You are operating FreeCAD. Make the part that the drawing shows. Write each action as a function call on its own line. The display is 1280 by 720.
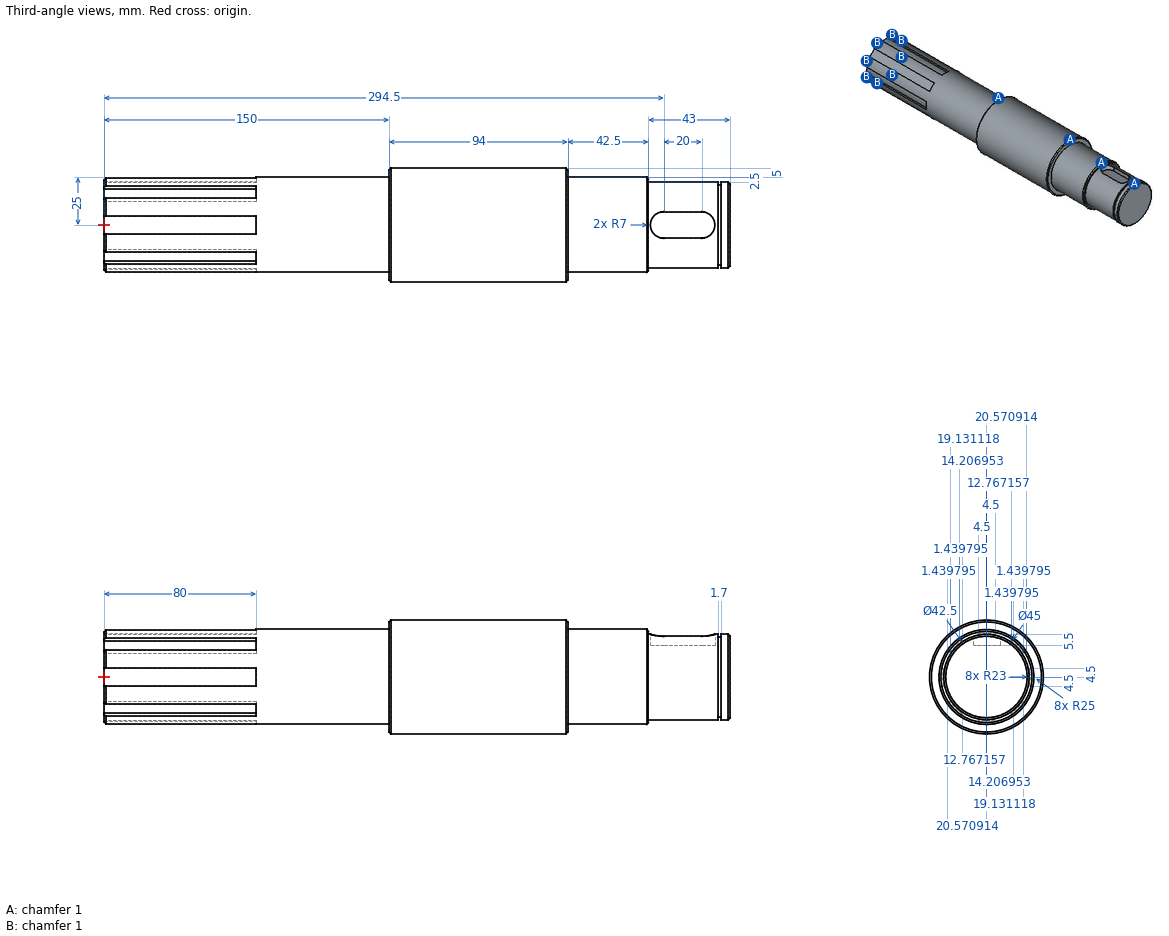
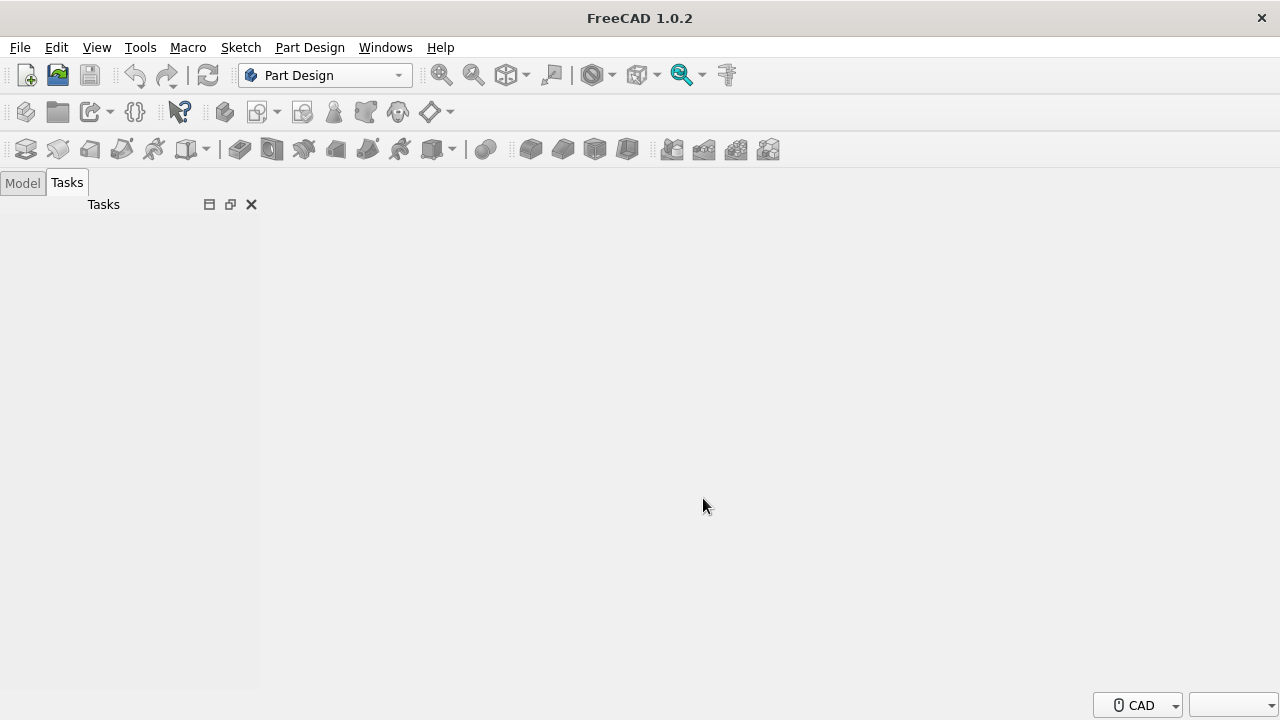
click(26, 76)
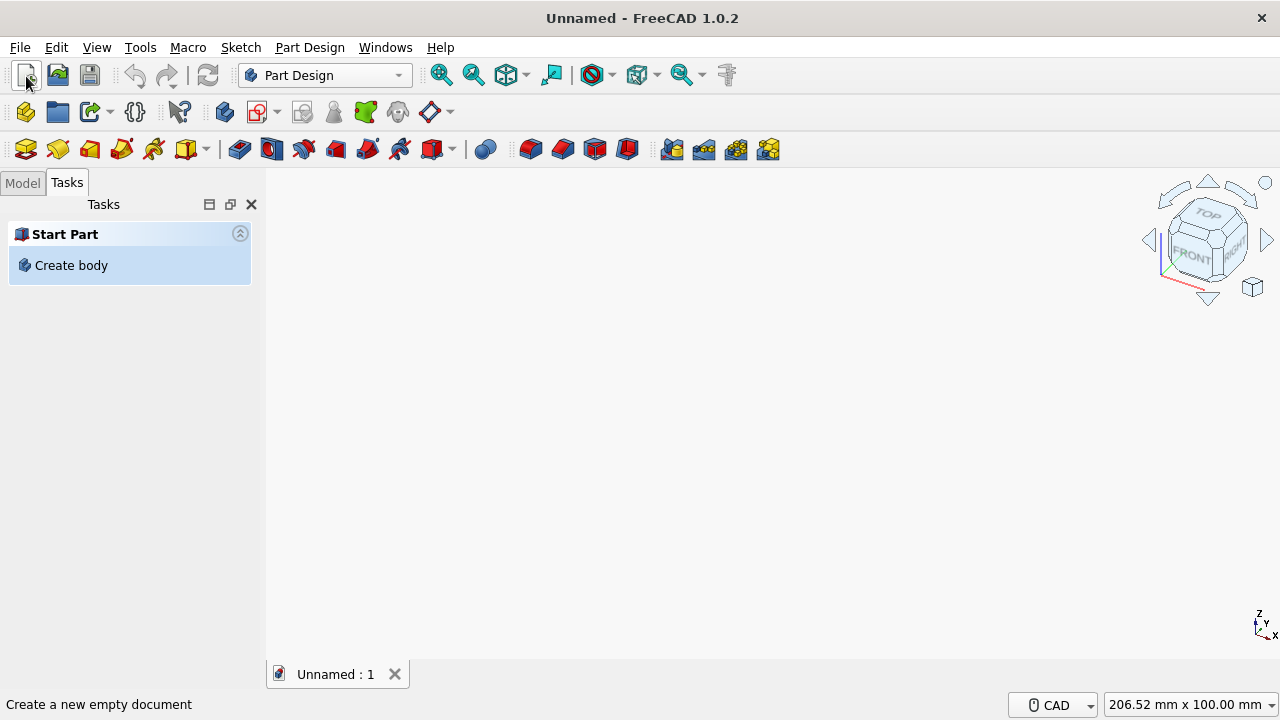
click(258, 112)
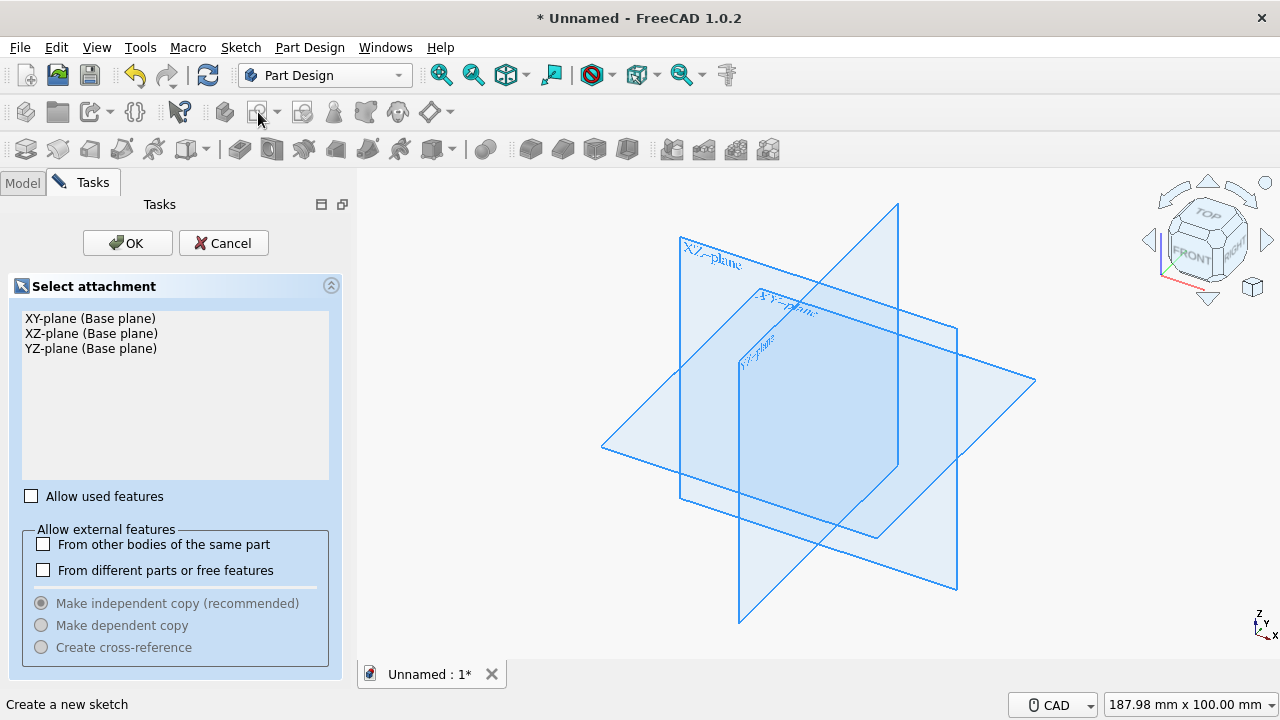
click(82, 318)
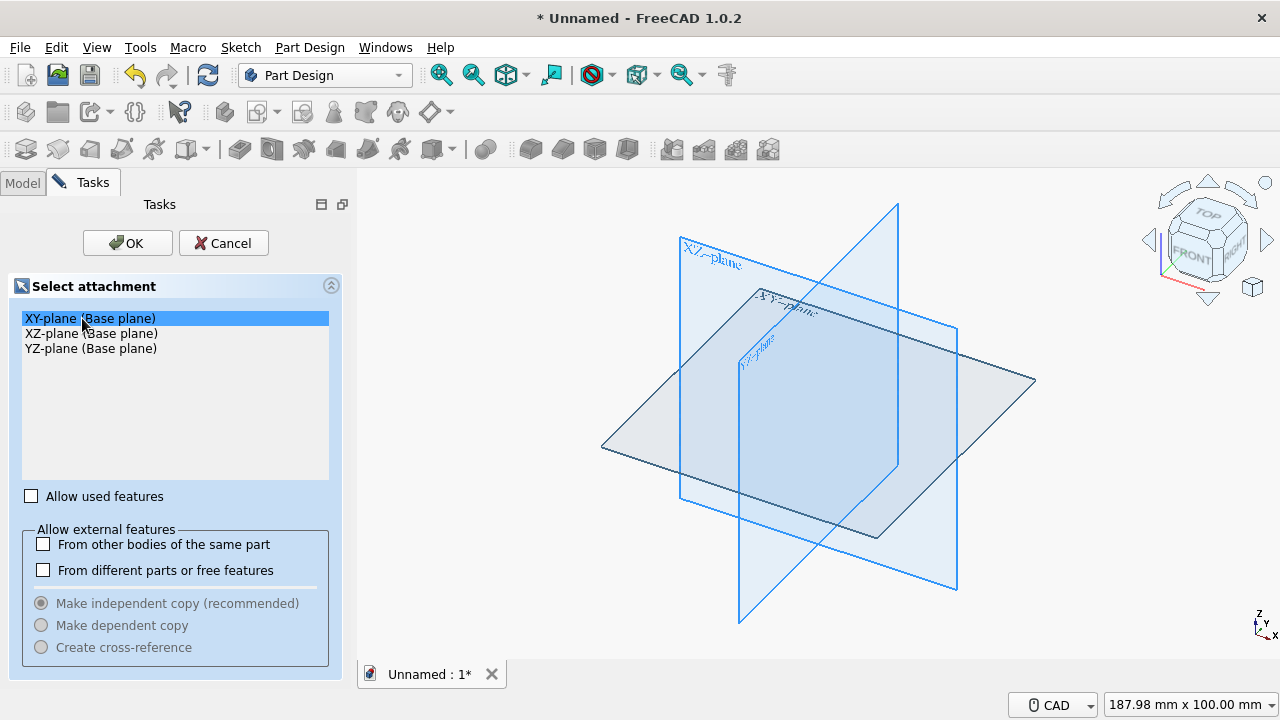
click(128, 243)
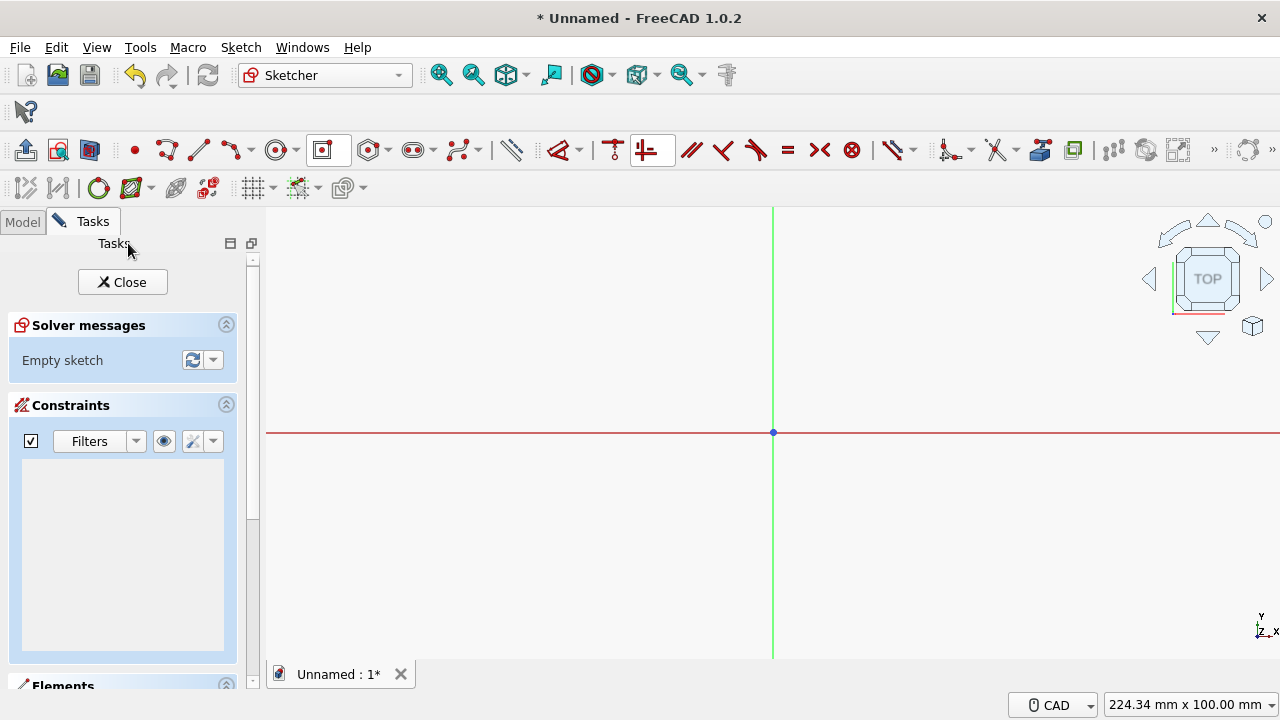
scroll(294, 472, down, 5)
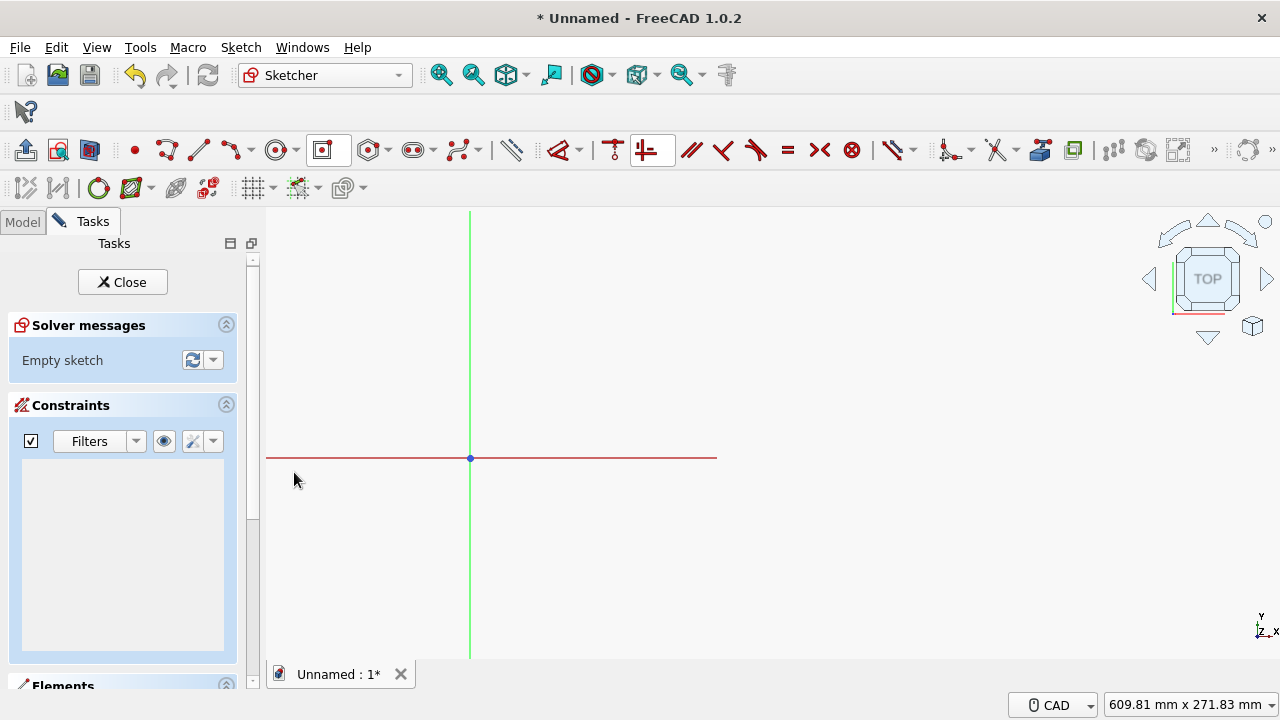
click(168, 150)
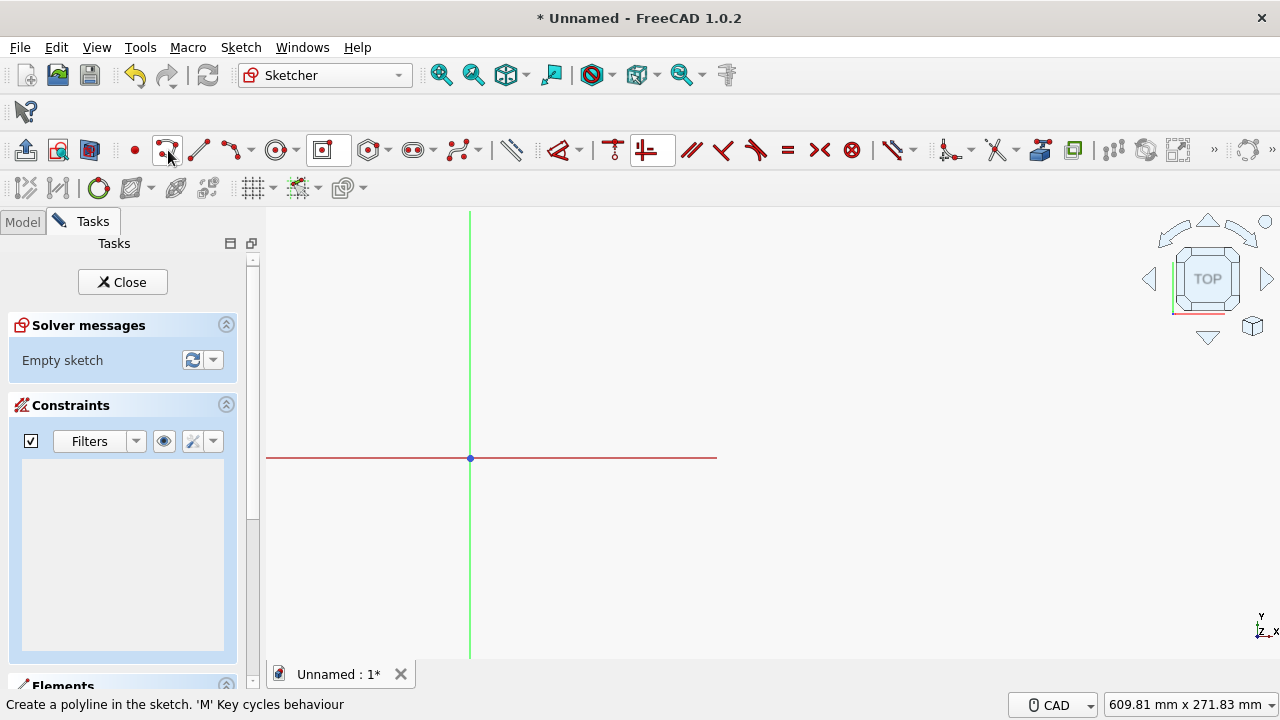
click(470, 458)
click(1018, 449)
click(1018, 421)
click(947, 421)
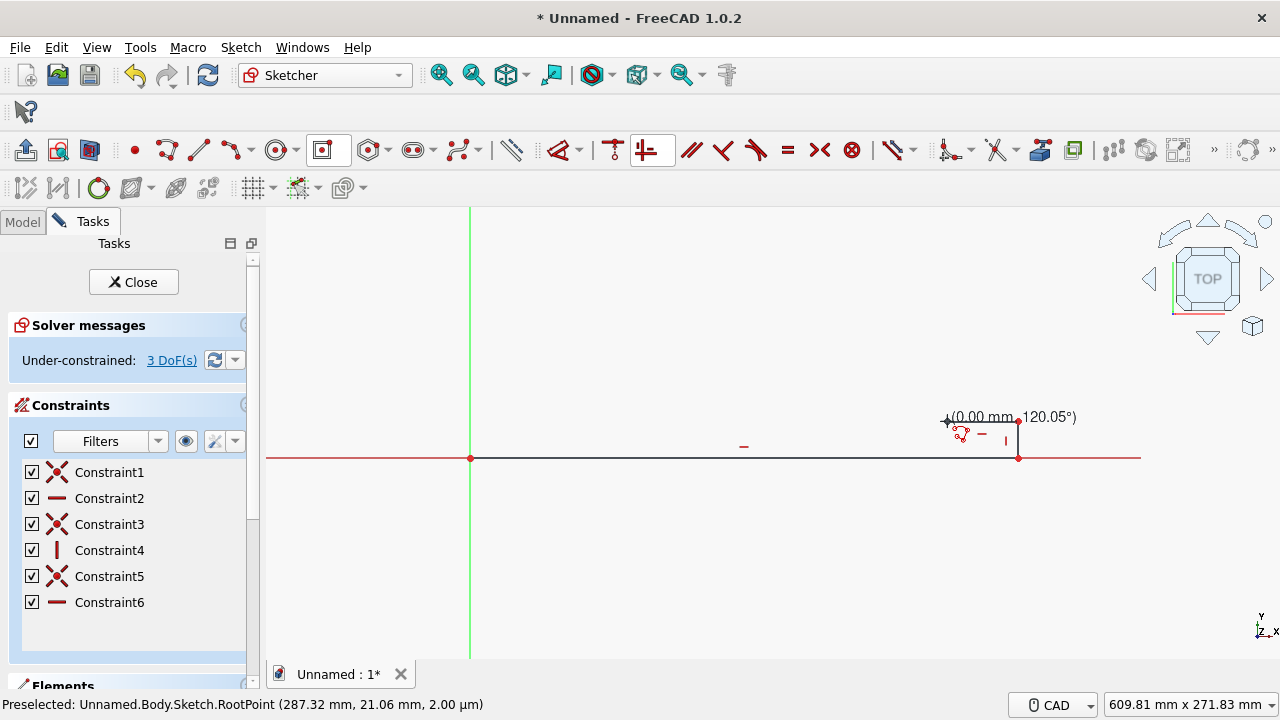
scroll(947, 416, up, 7)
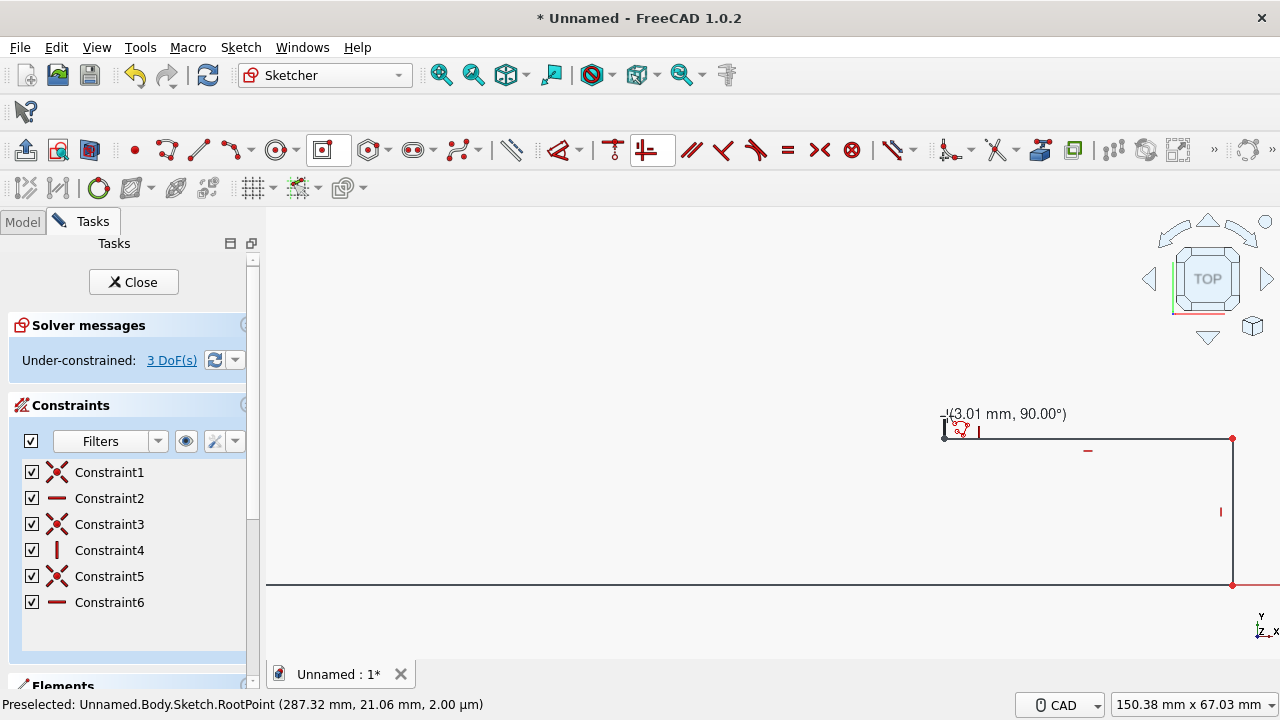
click(945, 416)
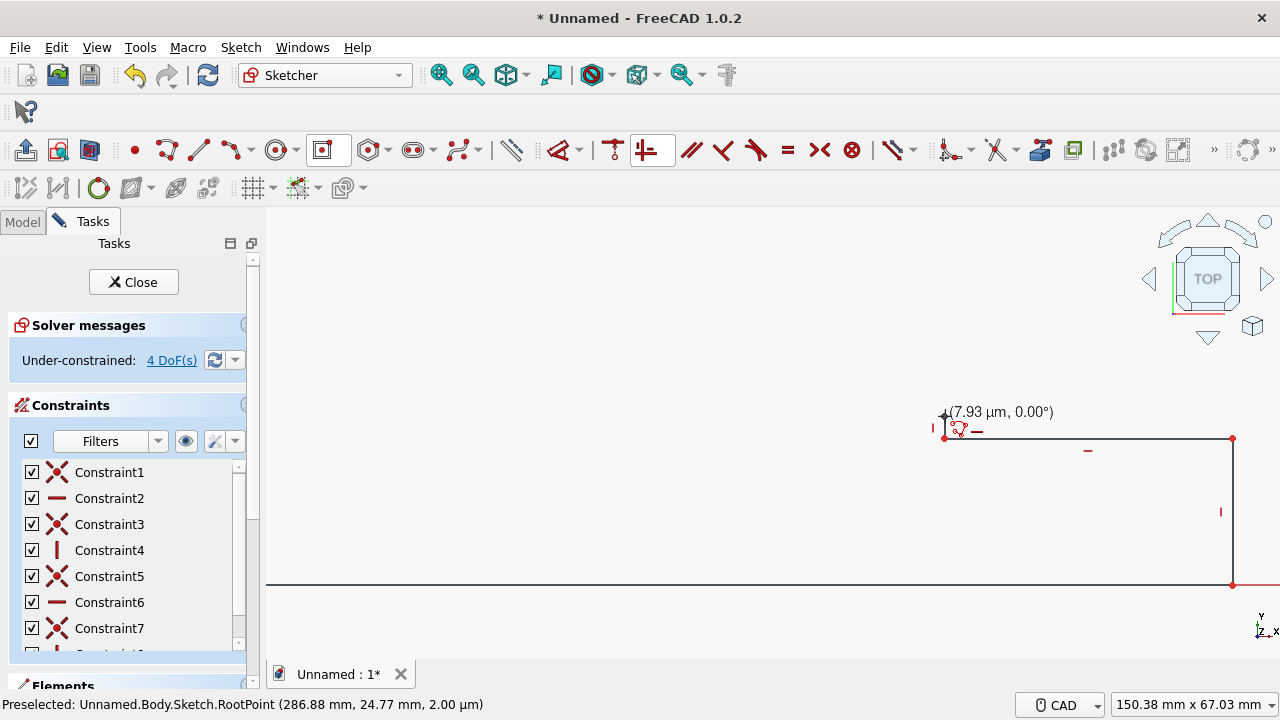
scroll(895, 416, down, 7)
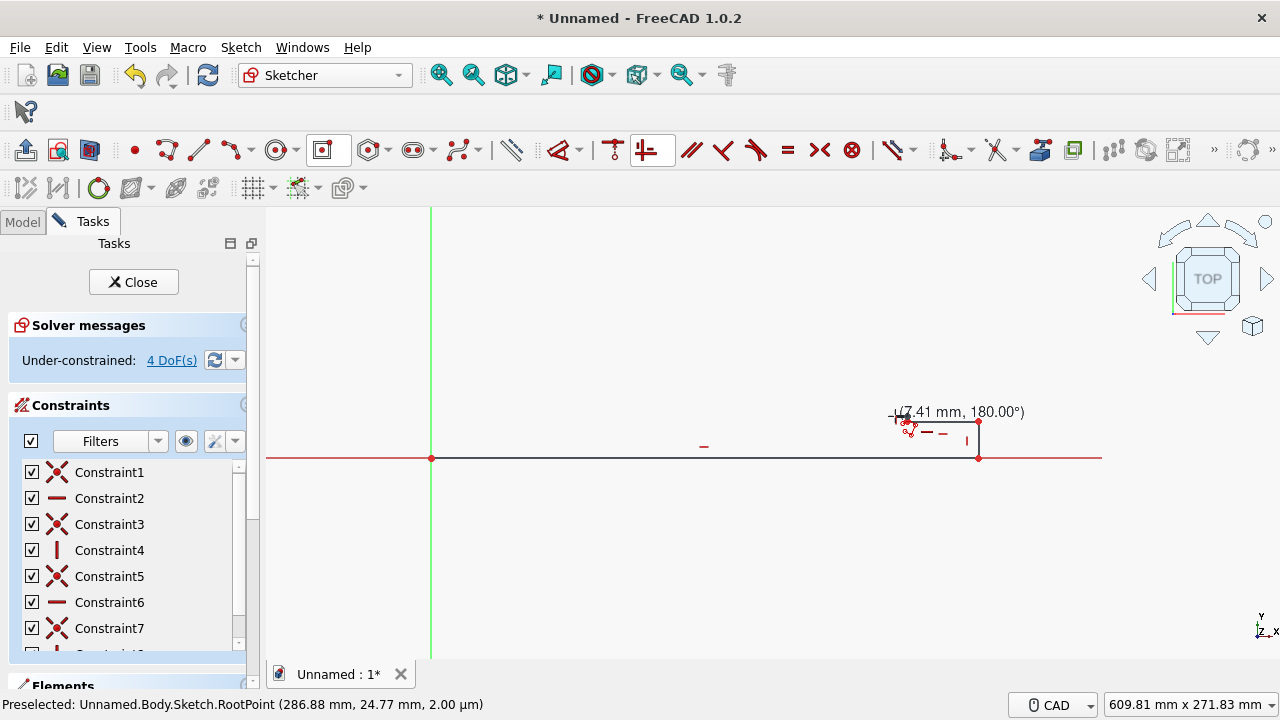
click(837, 416)